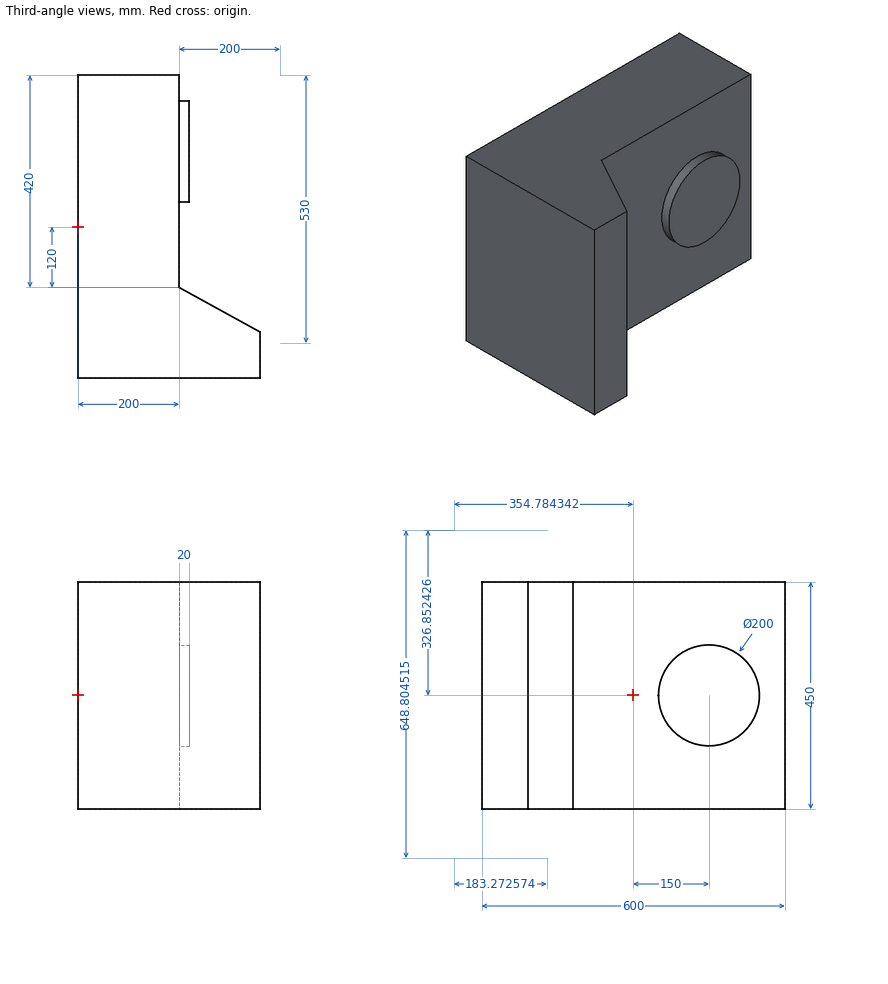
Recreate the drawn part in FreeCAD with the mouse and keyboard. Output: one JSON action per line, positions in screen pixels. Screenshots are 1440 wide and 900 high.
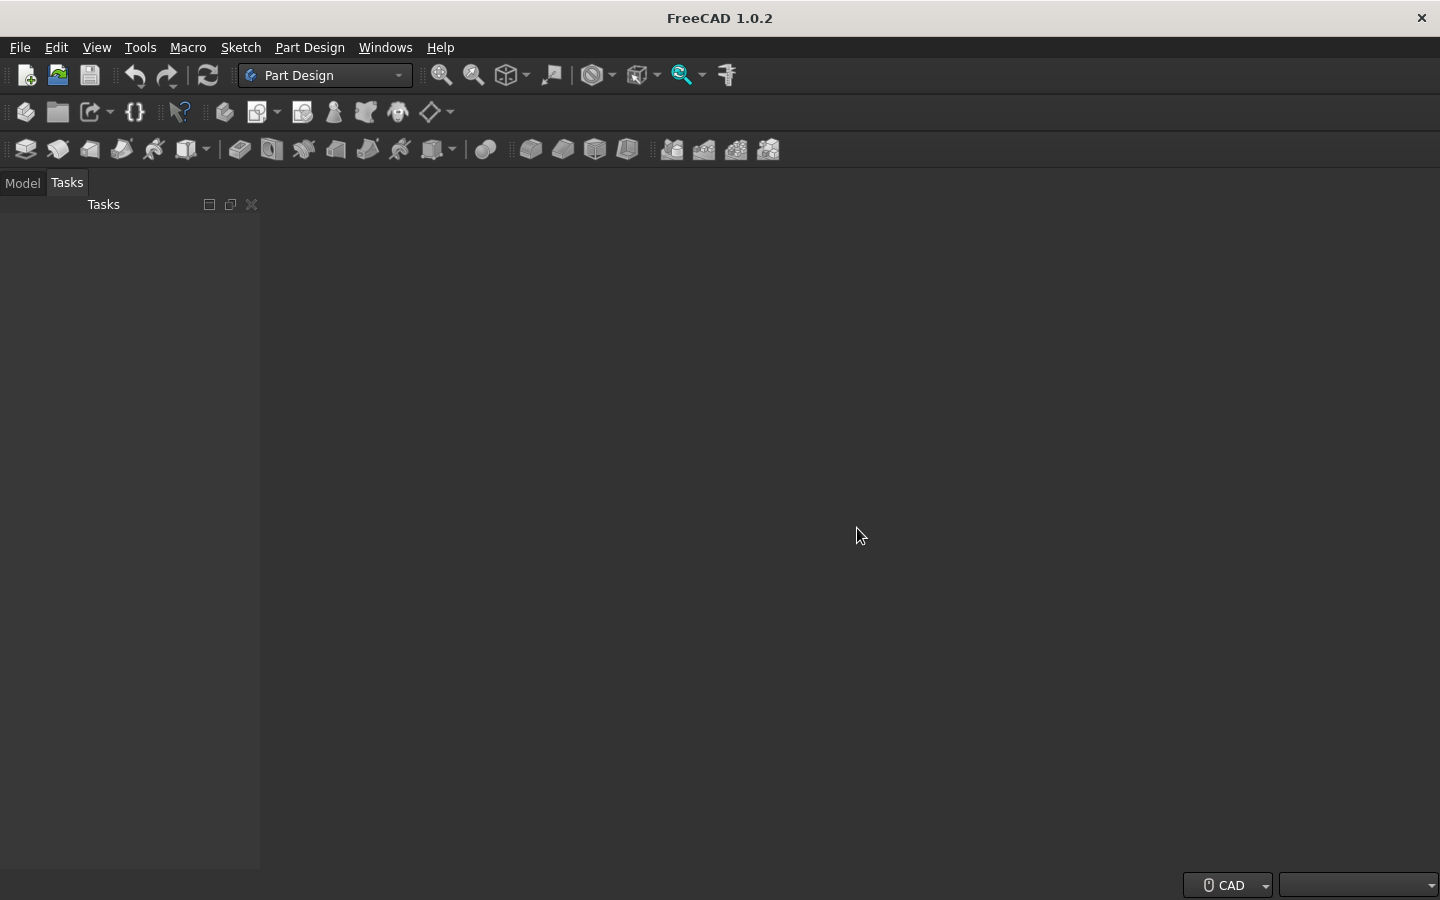
{"action": "key", "text": "ctrl+n"}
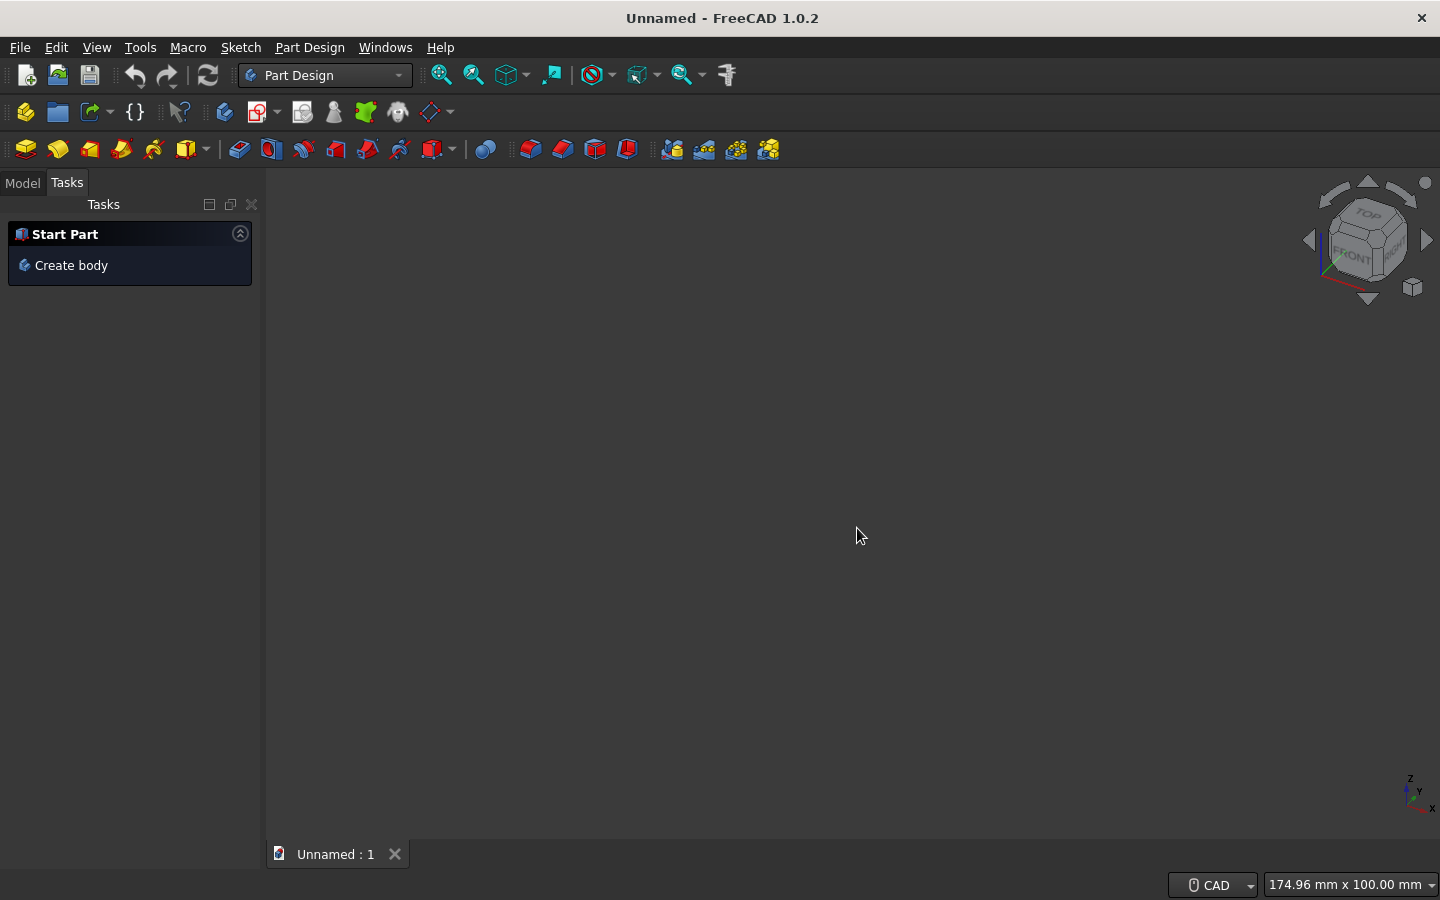
{"action": "left_click", "coordinate": [258, 112]}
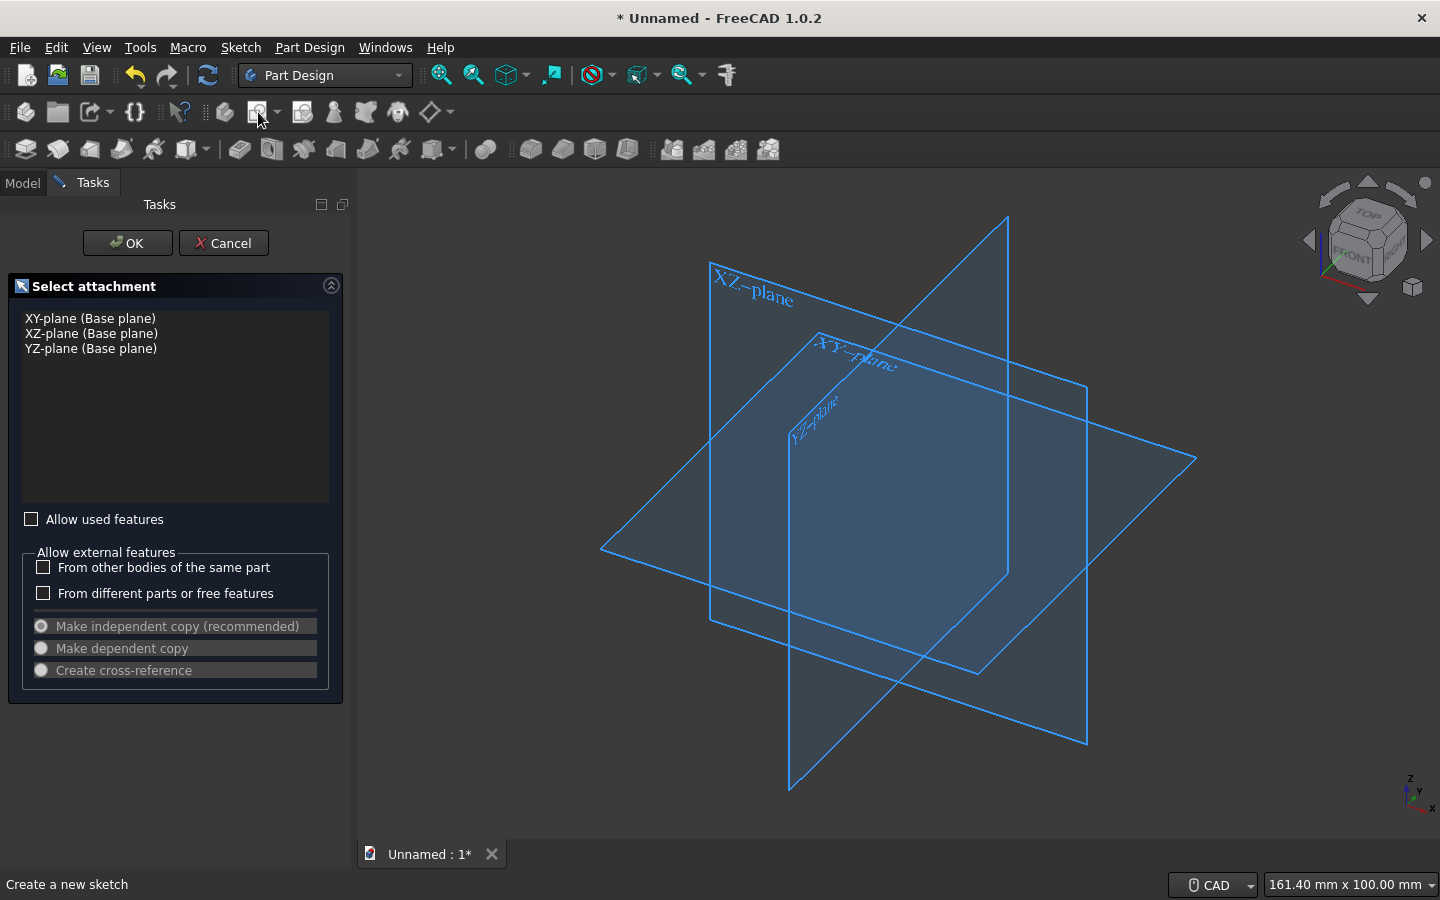
{"action": "left_click", "coordinate": [82, 348]}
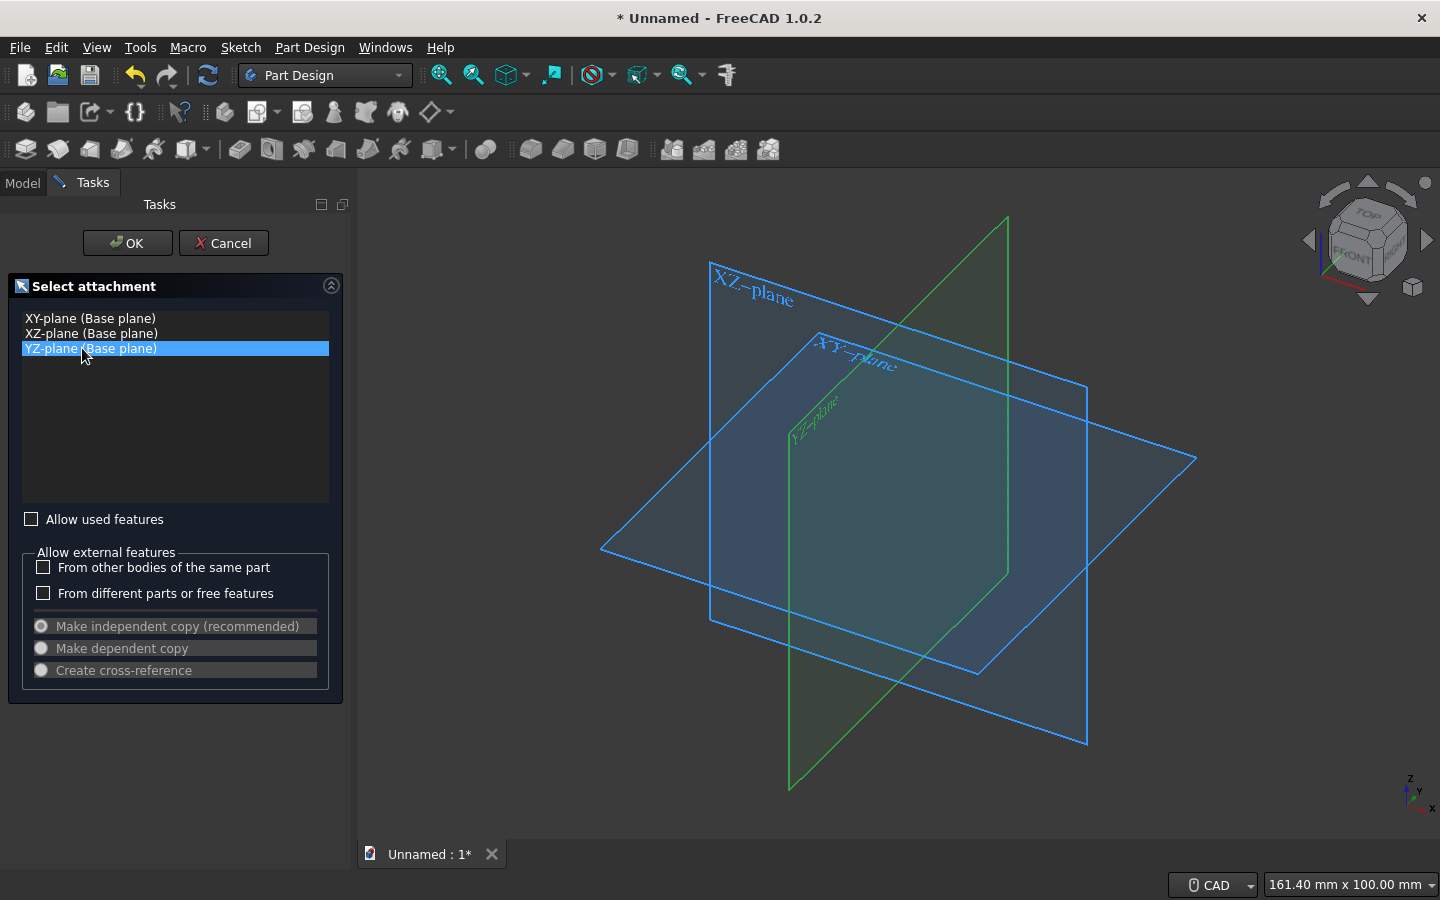
{"action": "left_click", "coordinate": [128, 243]}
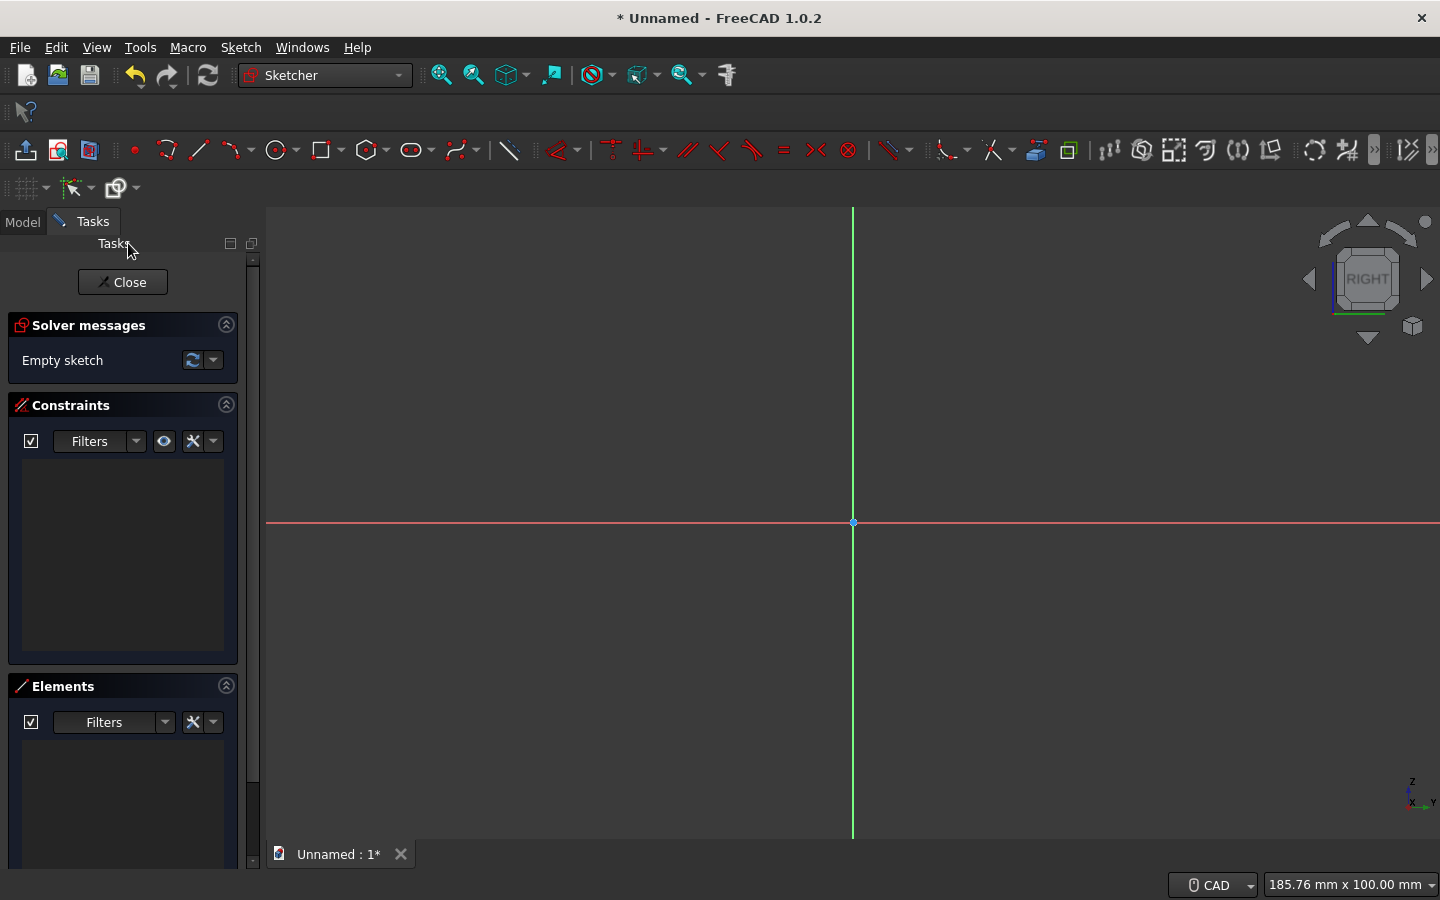
{"action": "scroll", "coordinate": [774, 523], "scroll_direction": "down", "scroll_amount": 10}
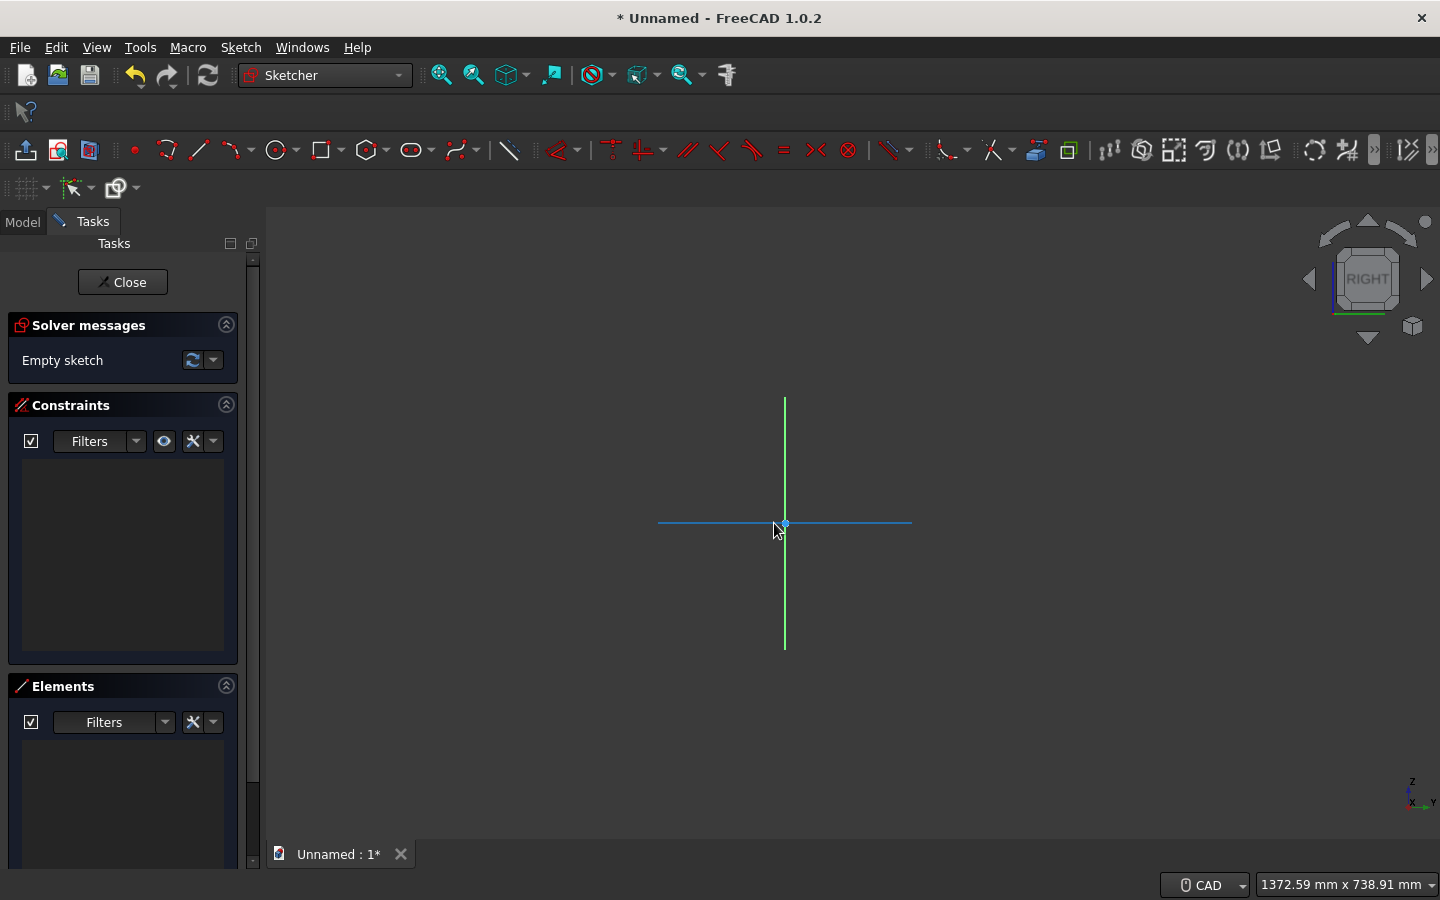
{"action": "left_click", "coordinate": [344, 150]}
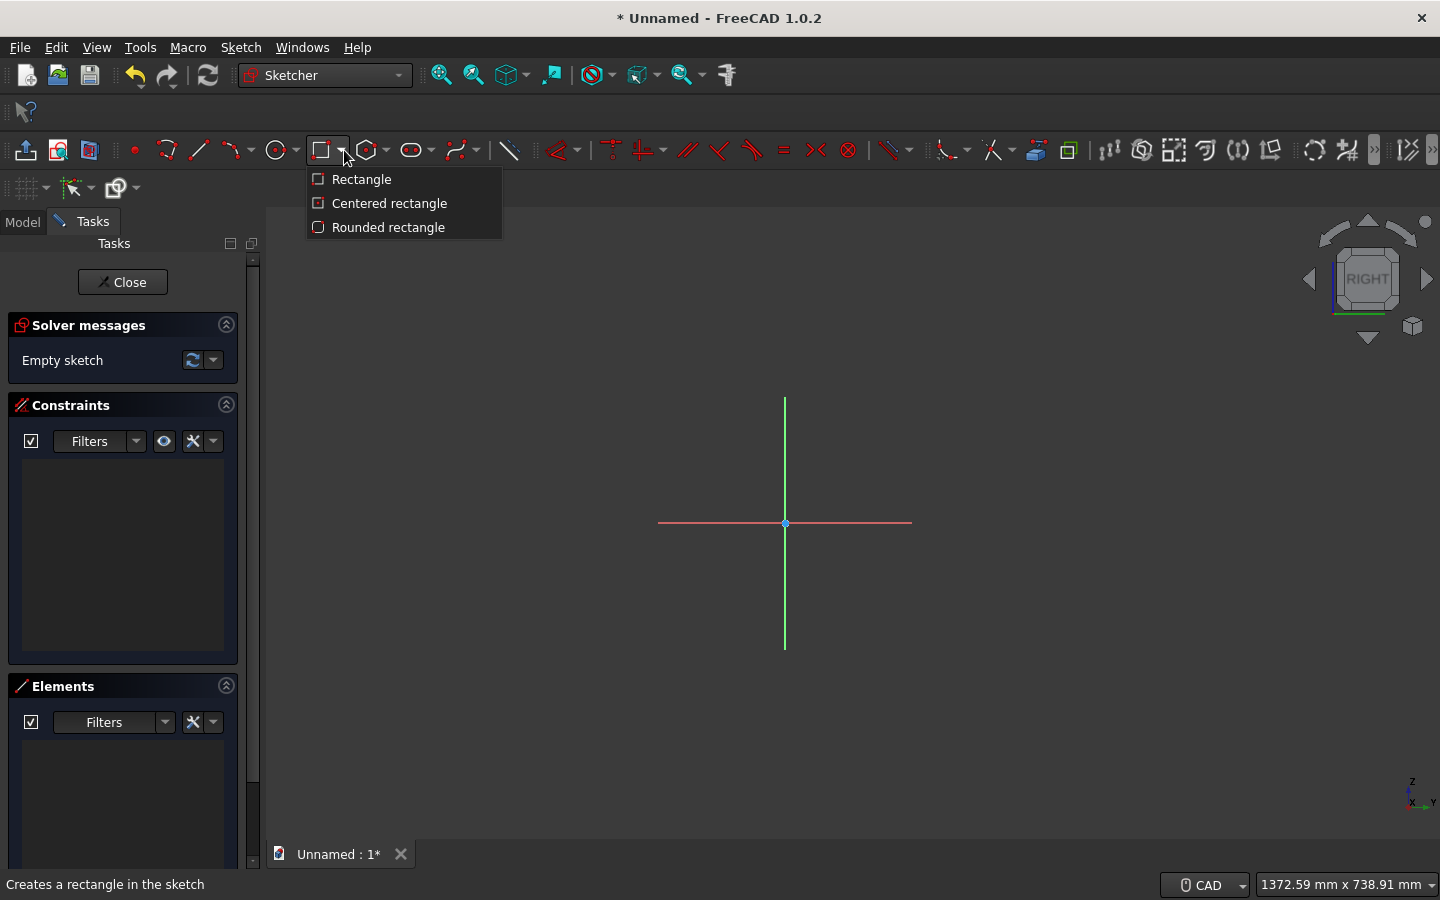
{"action": "left_click", "coordinate": [404, 203]}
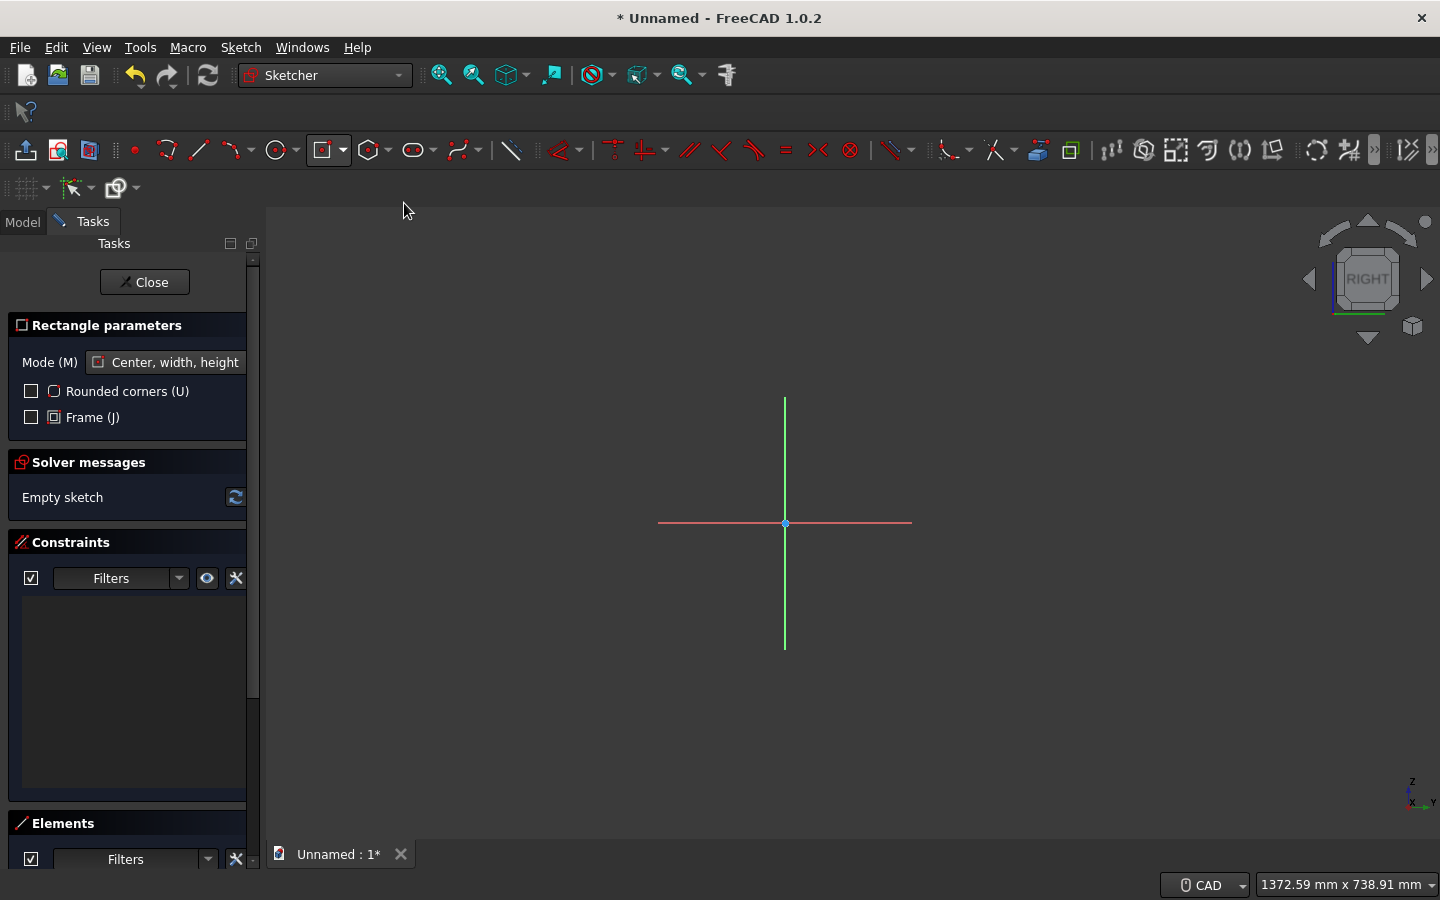
{"action": "left_click", "coordinate": [785, 523]}
{"action": "mouse_move", "coordinate": [1042, 331]}